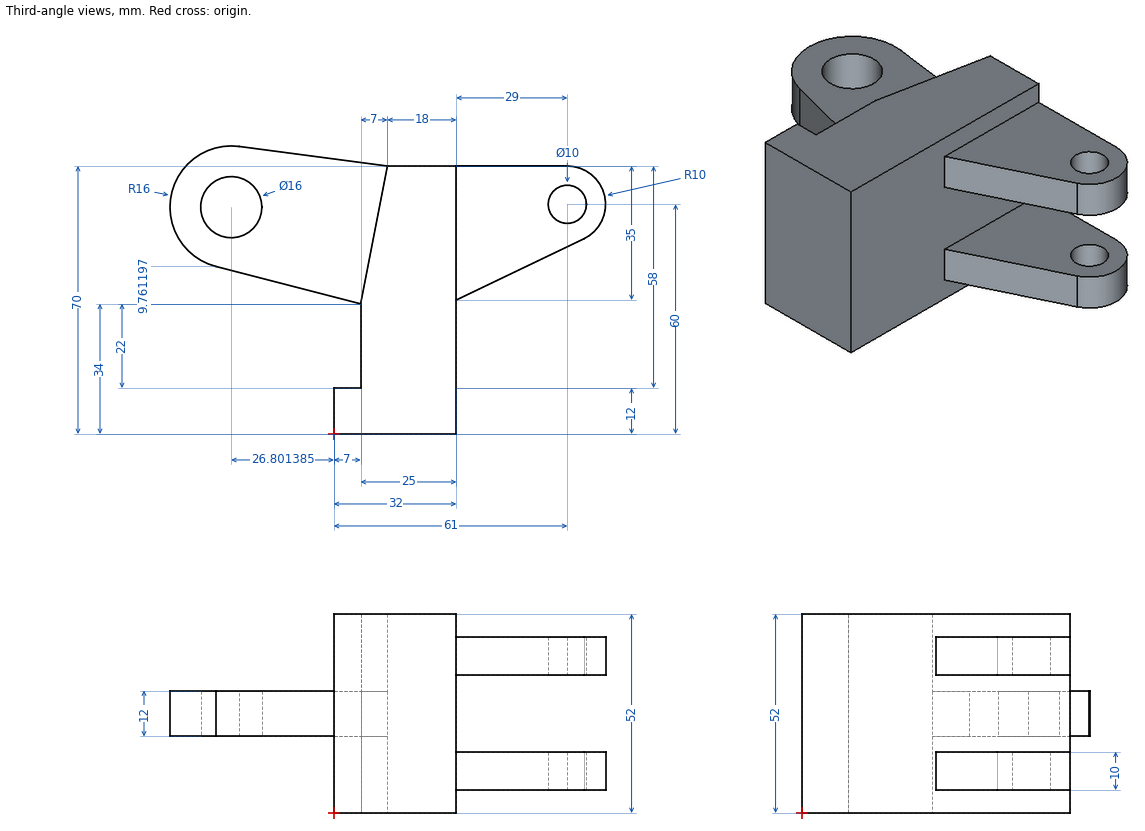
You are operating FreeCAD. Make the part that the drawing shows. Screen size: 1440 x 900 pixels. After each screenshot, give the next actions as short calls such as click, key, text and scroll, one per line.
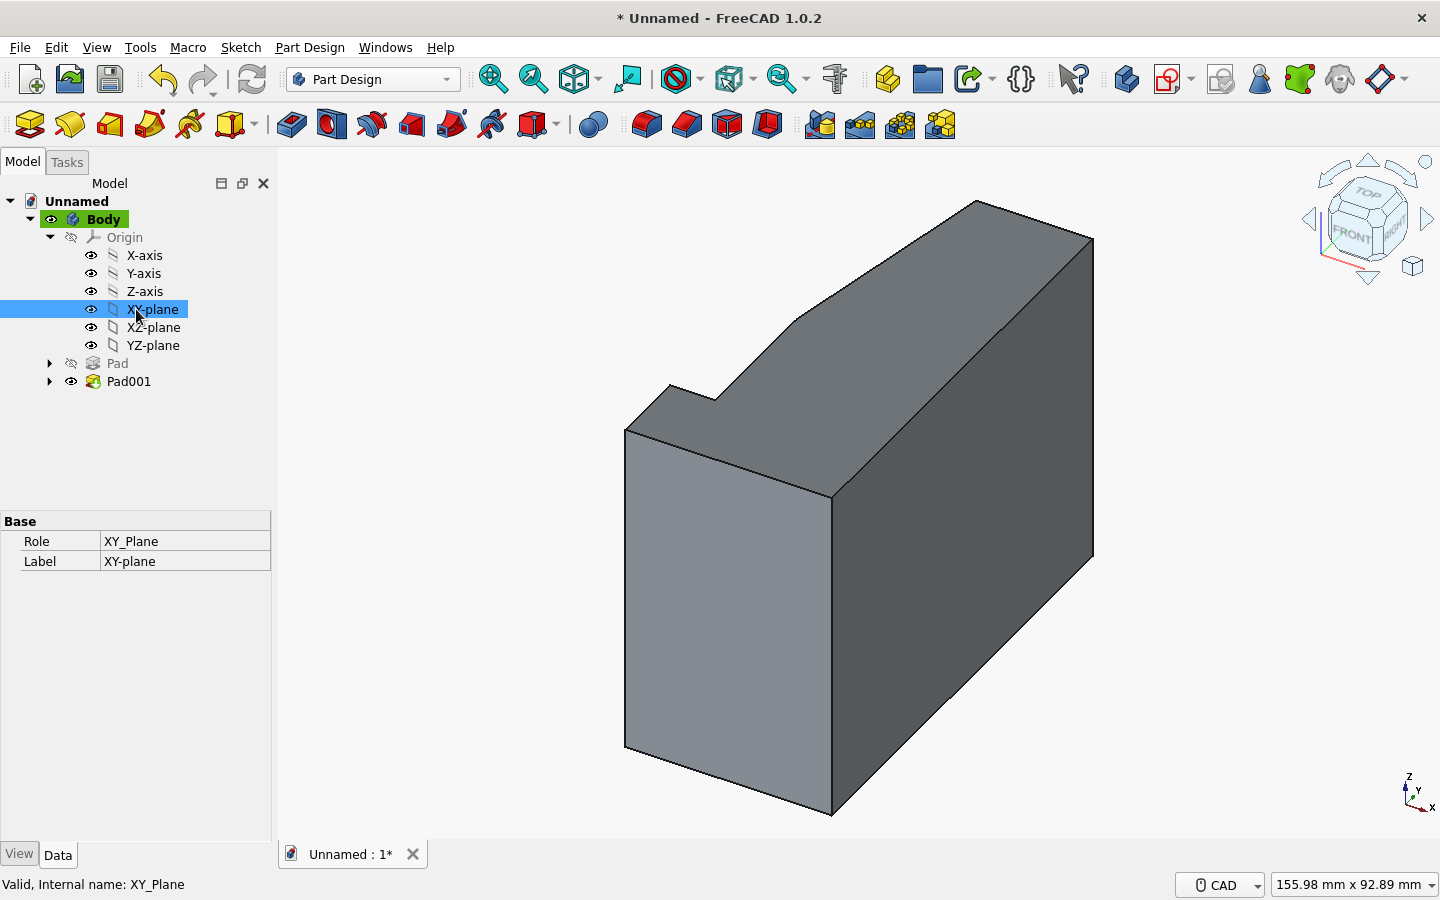
click(1380, 80)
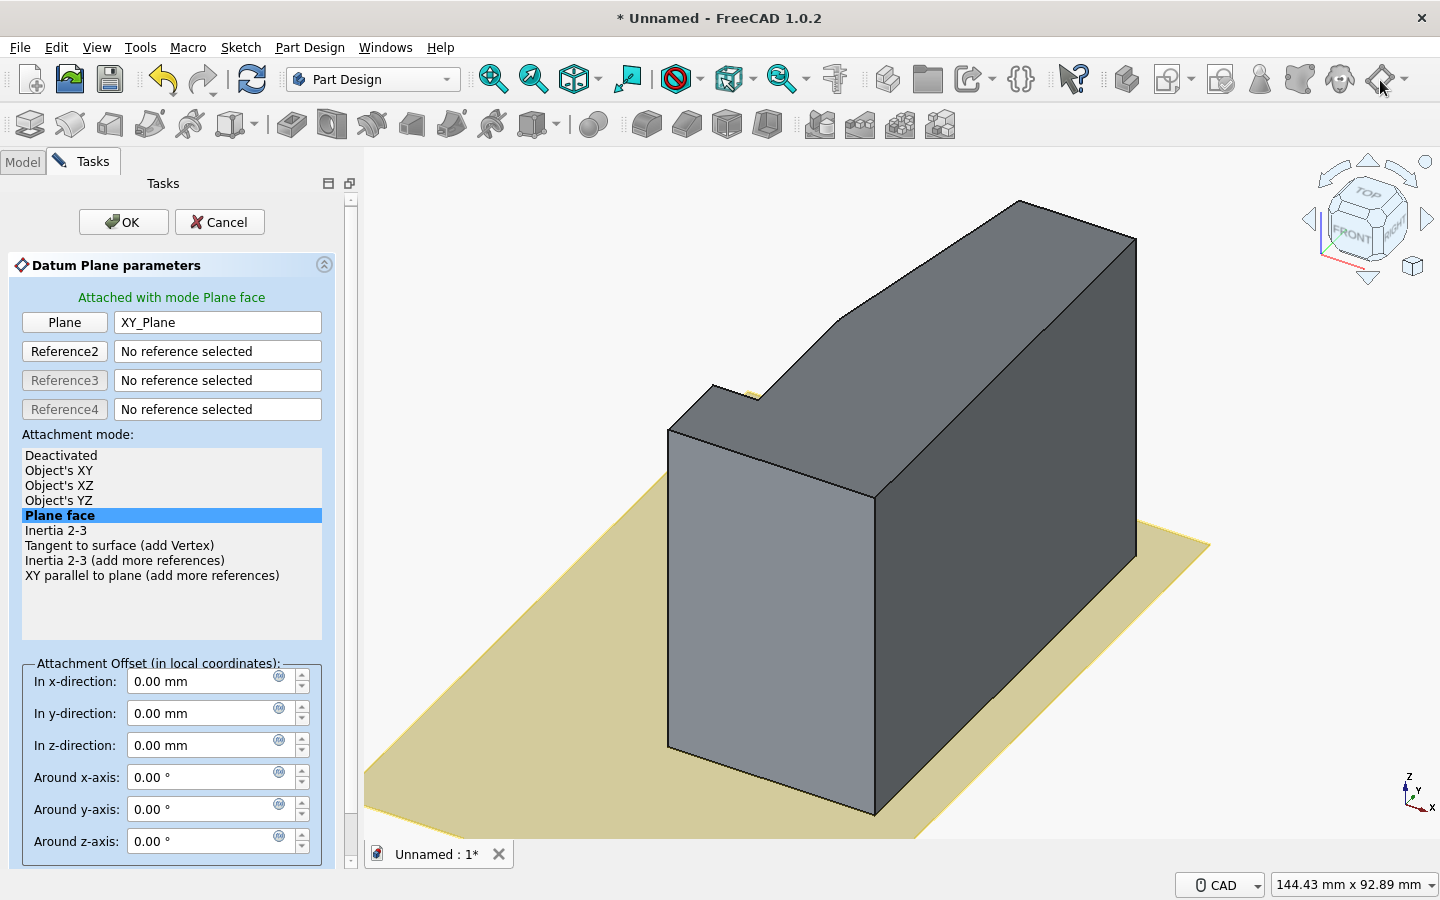
triple_click(210, 745)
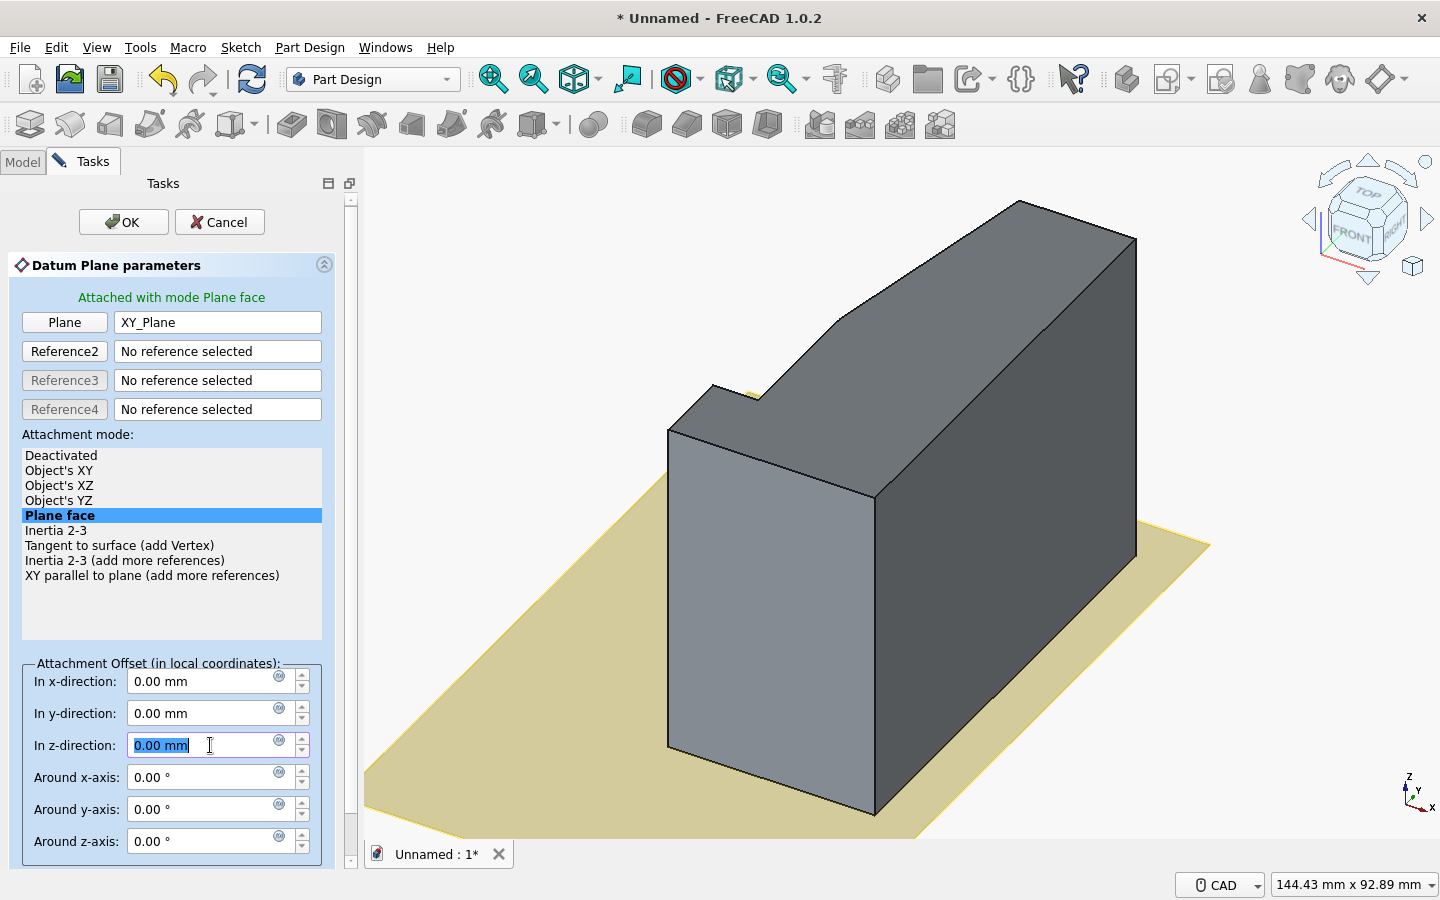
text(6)
key(Tab)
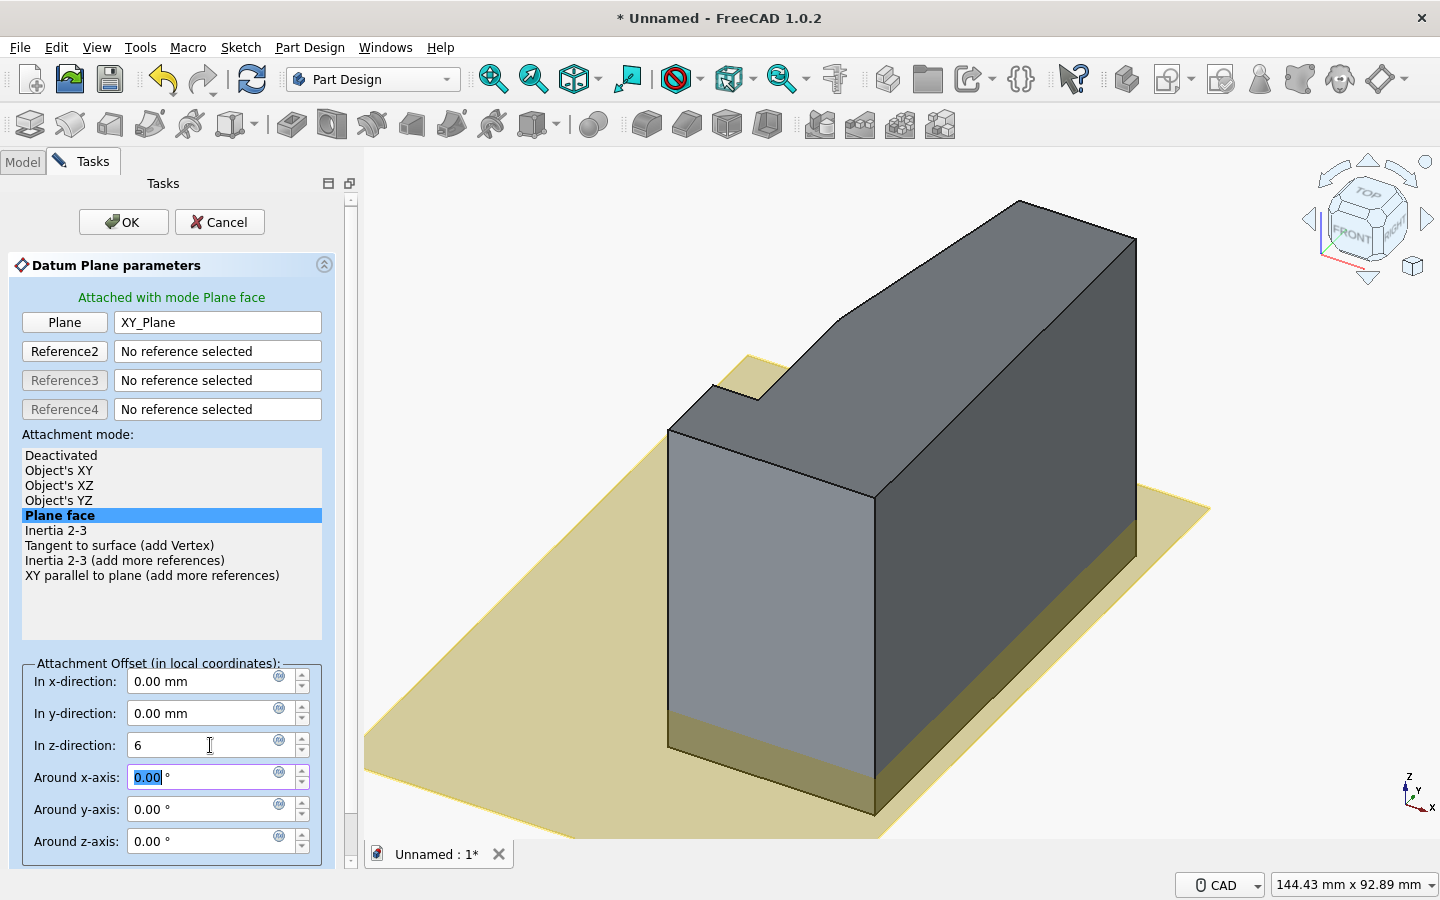
click(124, 222)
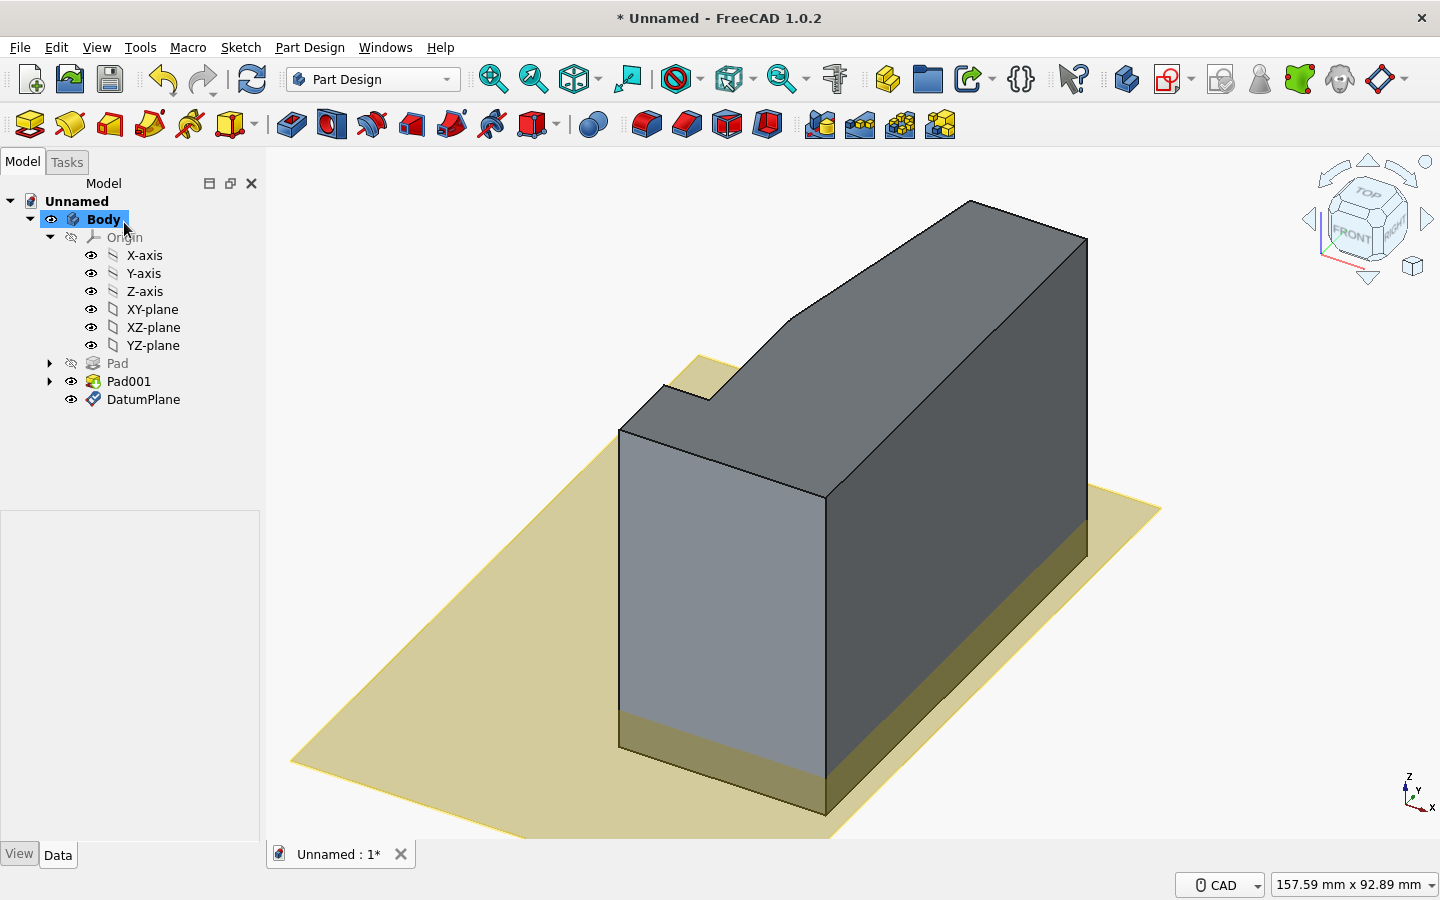
click(116, 399)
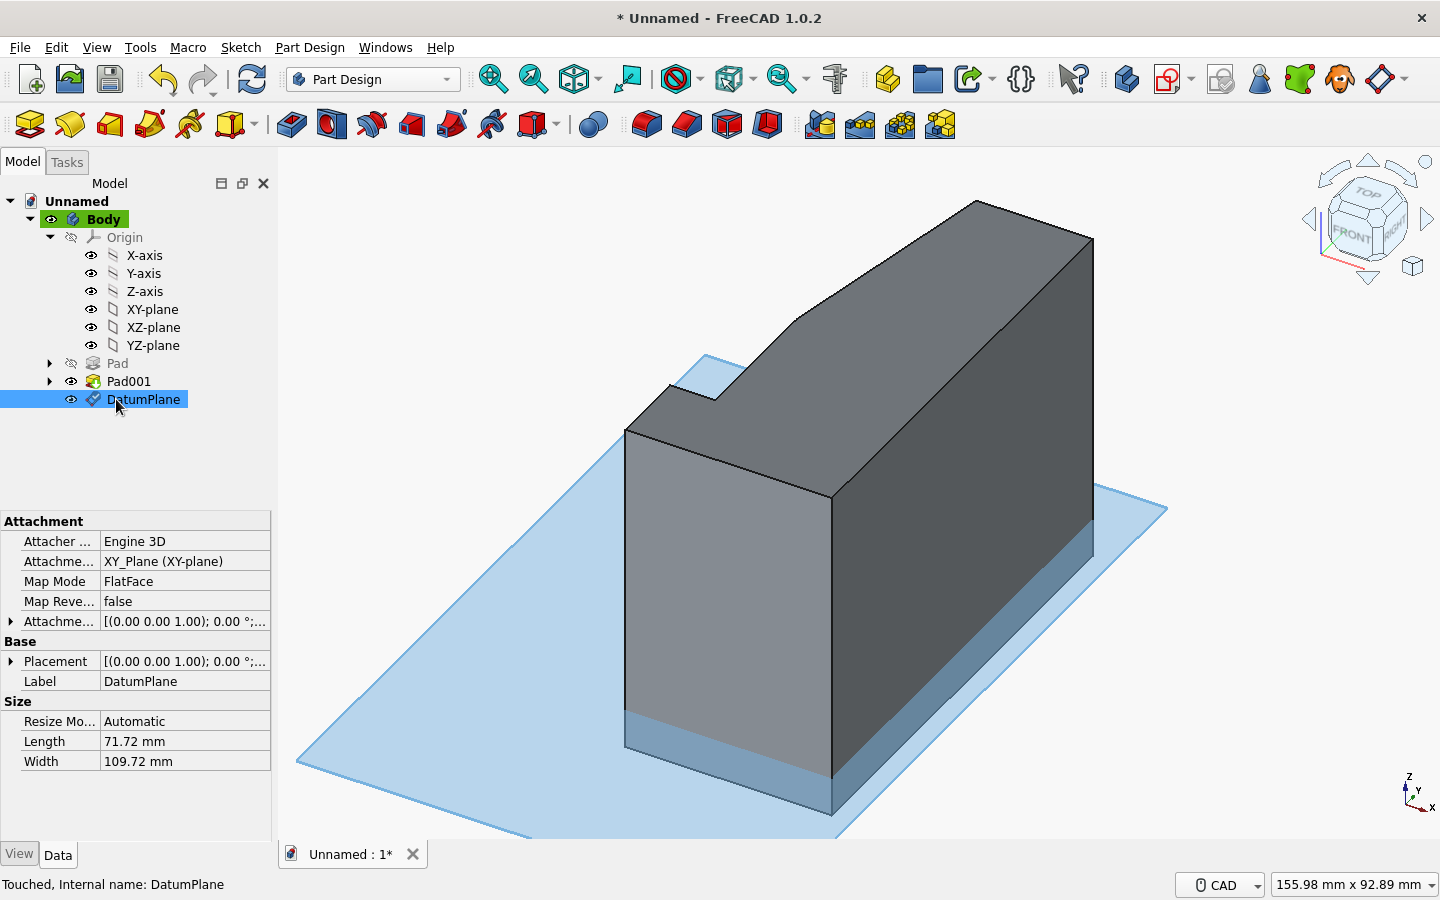
click(1168, 80)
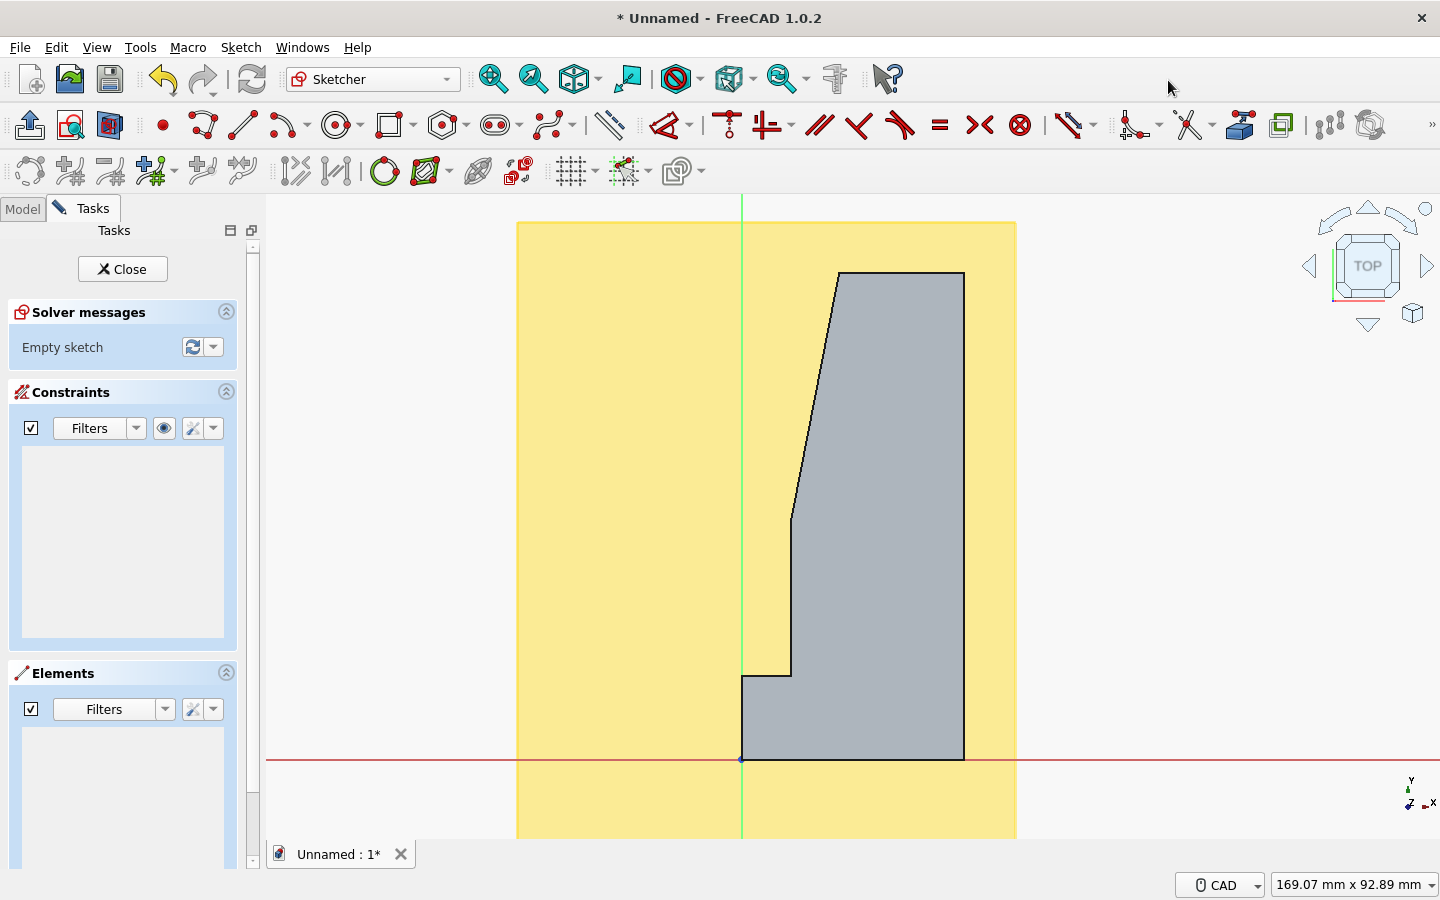
key(q)
key(s)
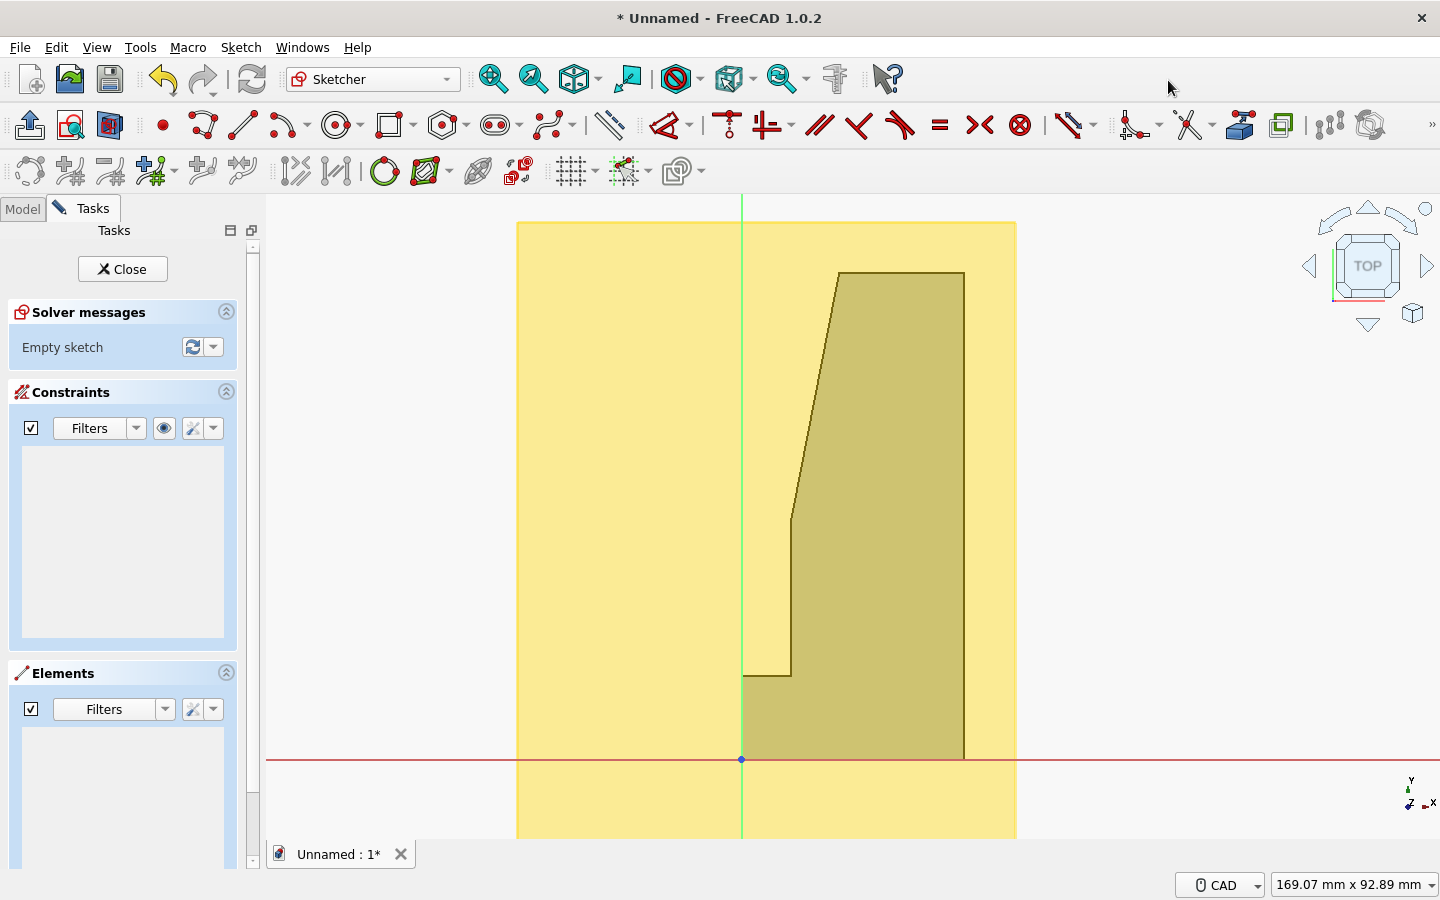
click(204, 126)